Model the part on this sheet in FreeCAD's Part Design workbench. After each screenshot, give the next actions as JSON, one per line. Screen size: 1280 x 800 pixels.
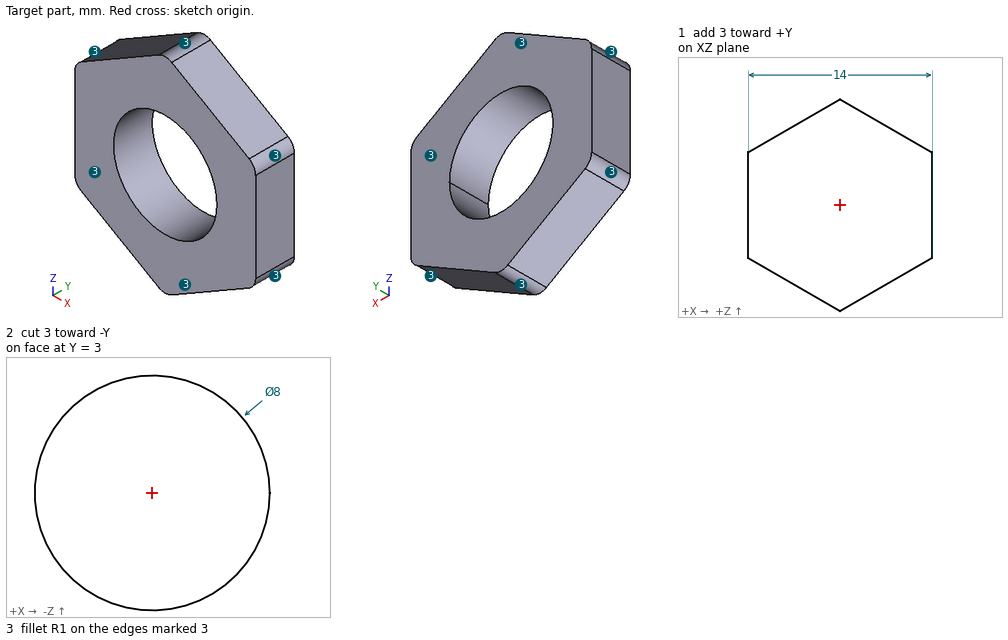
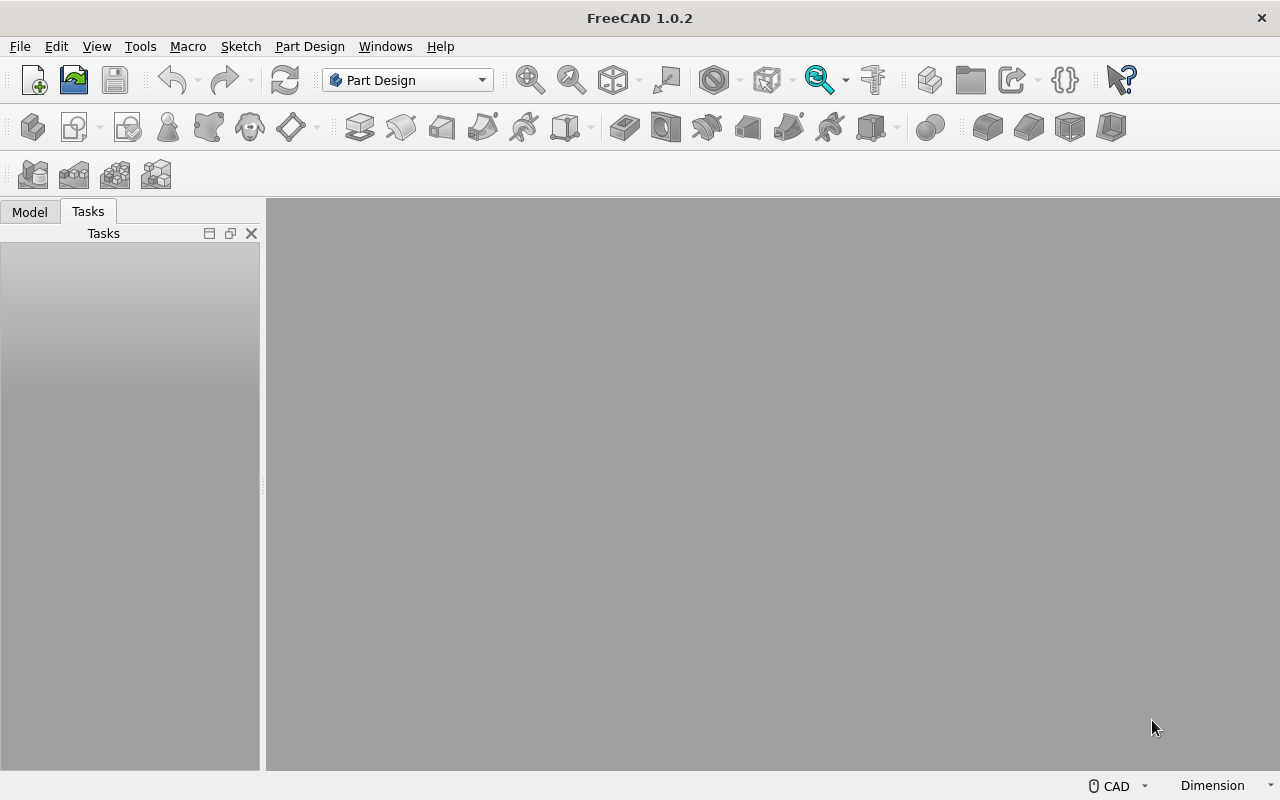
{"action": "key", "text": "ctrl+n"}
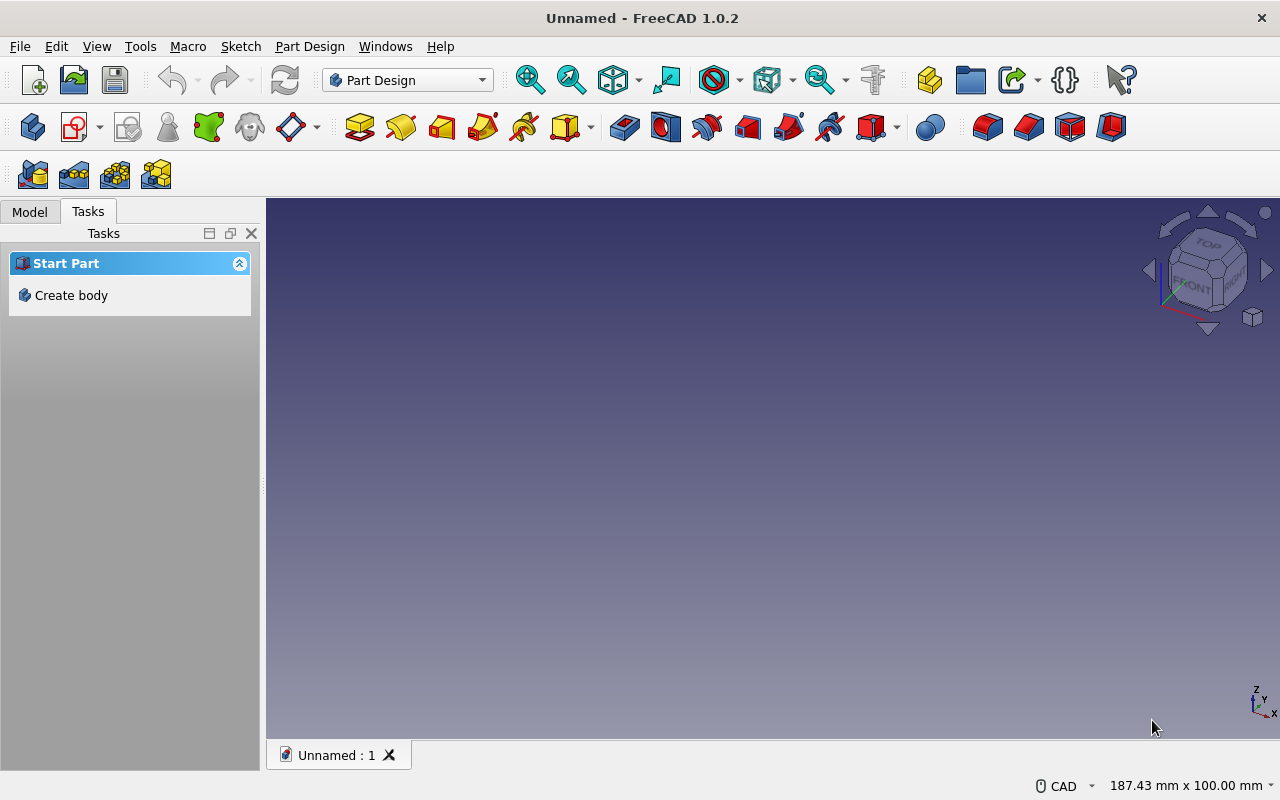
{"action": "left_click", "coordinate": [74, 128]}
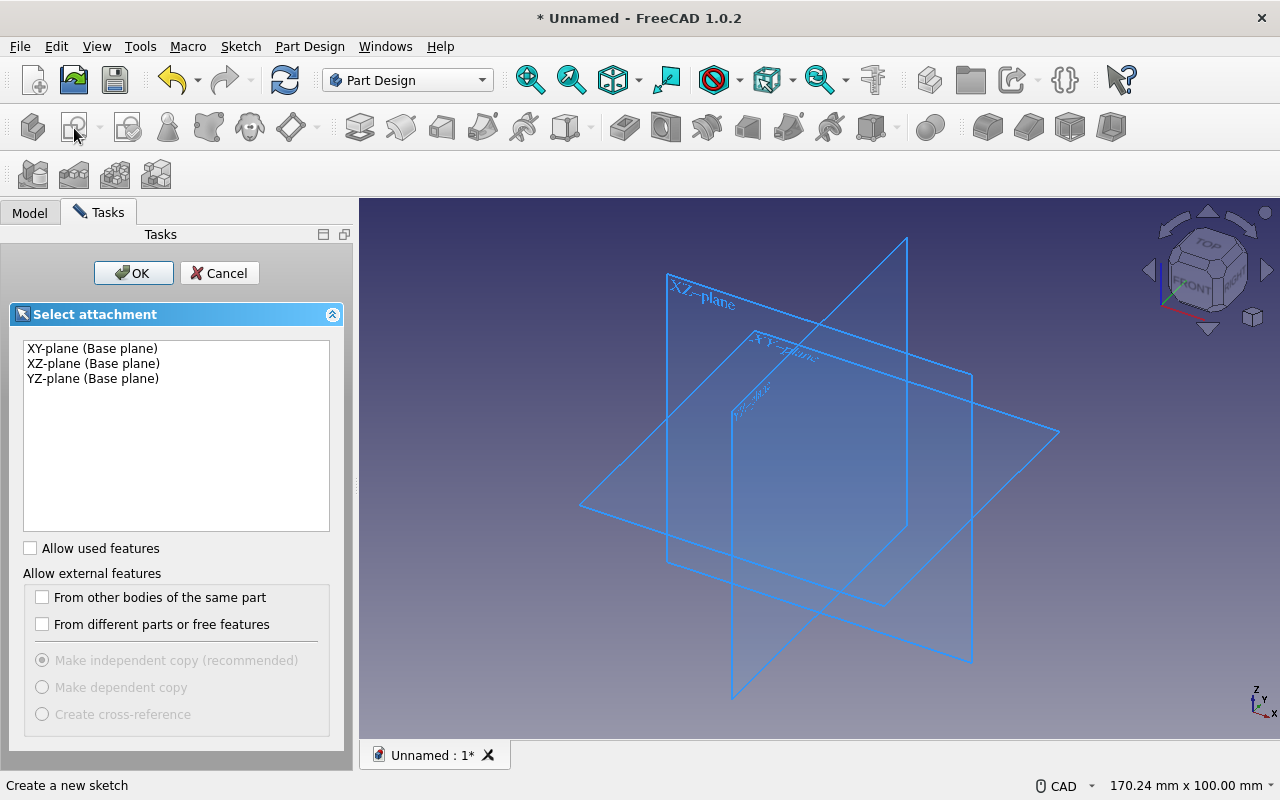
{"action": "left_click", "coordinate": [84, 364]}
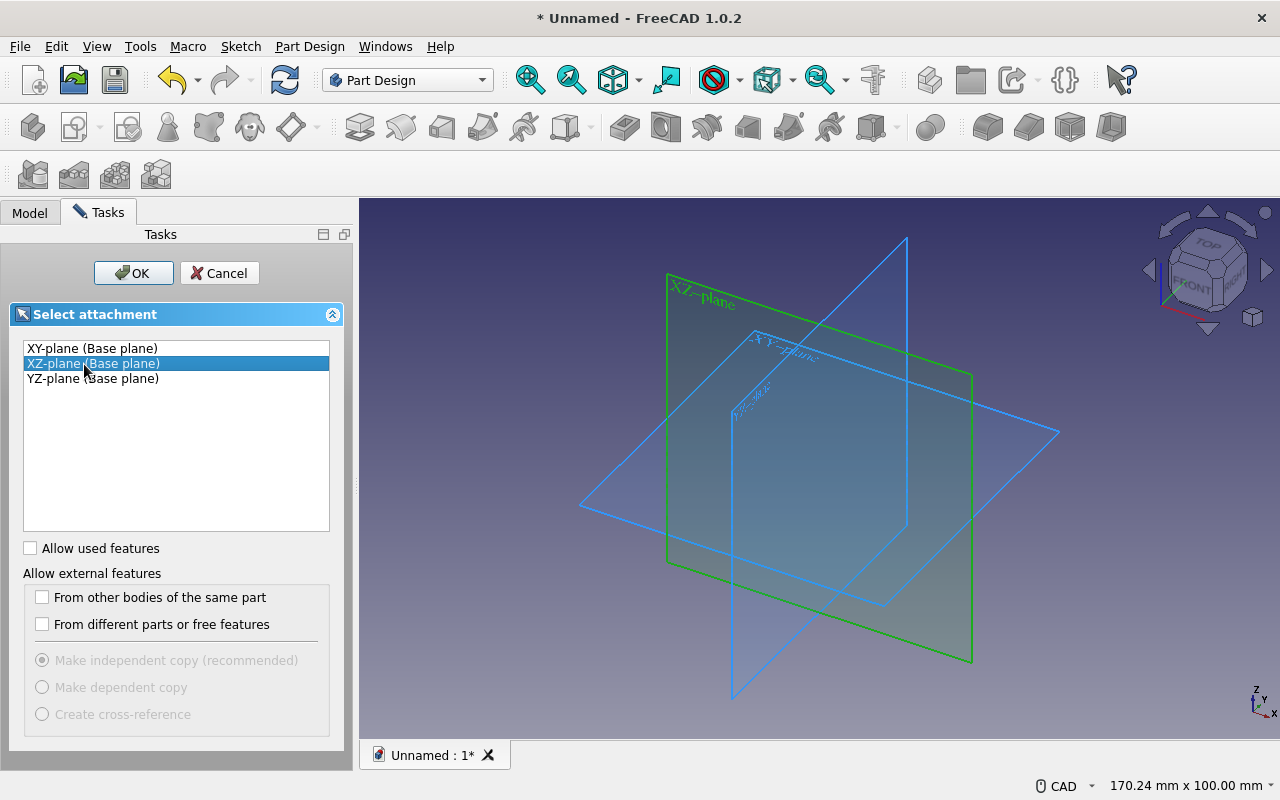
{"action": "left_click", "coordinate": [134, 273]}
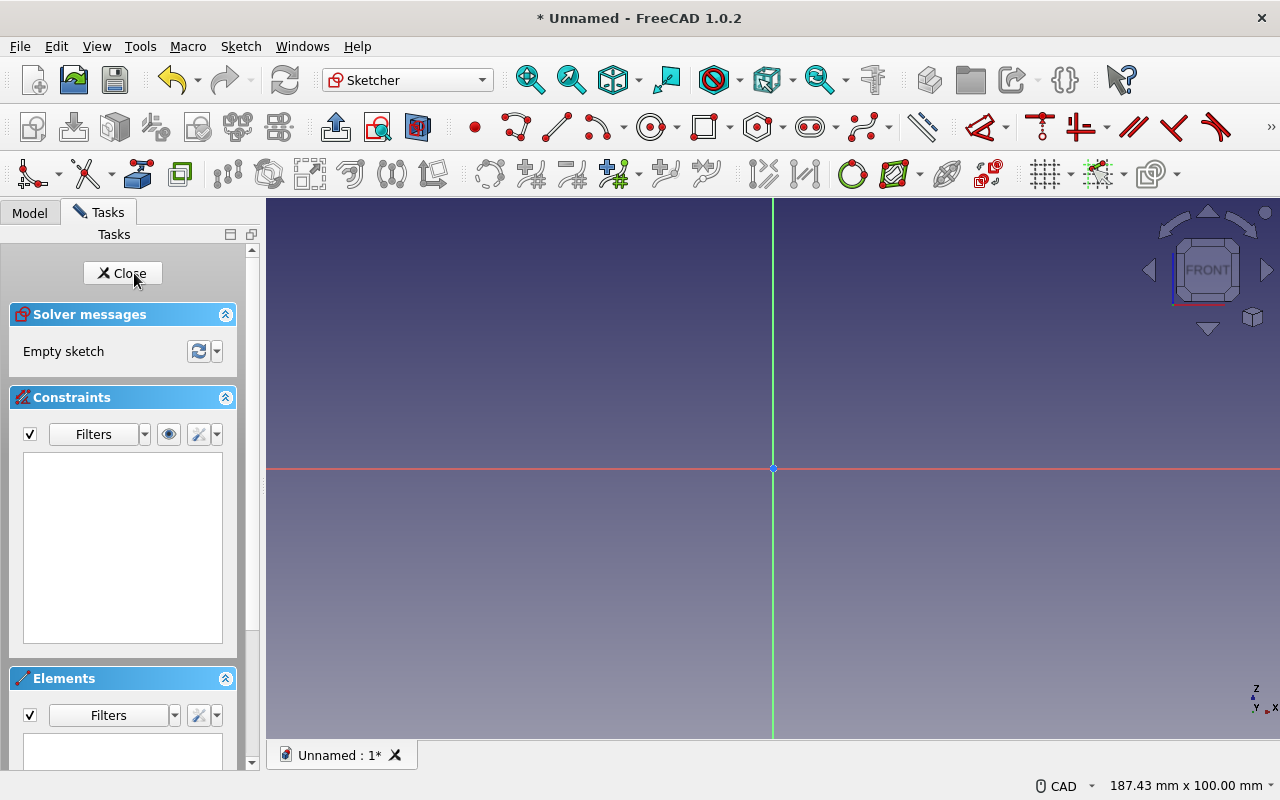
{"action": "scroll", "coordinate": [795, 468], "scroll_direction": "up", "scroll_amount": 7}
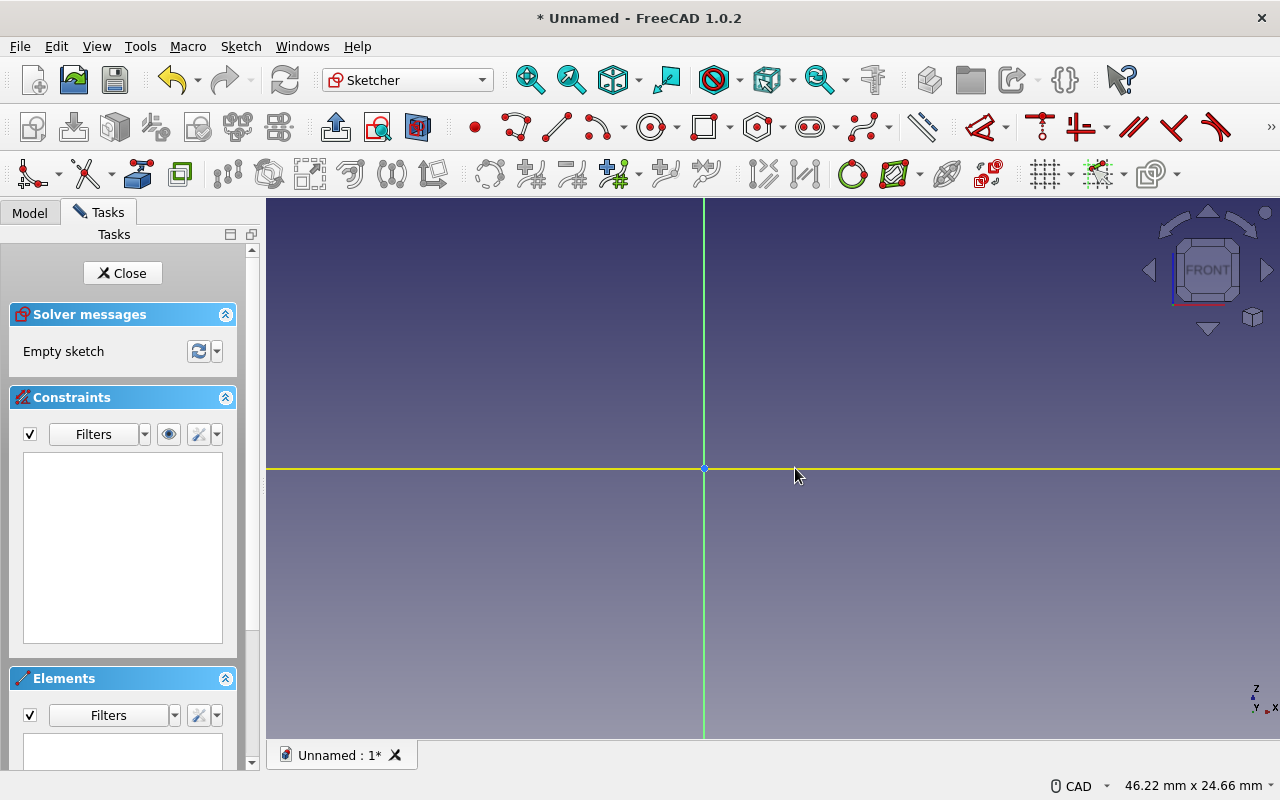
{"action": "key", "text": "g p 6"}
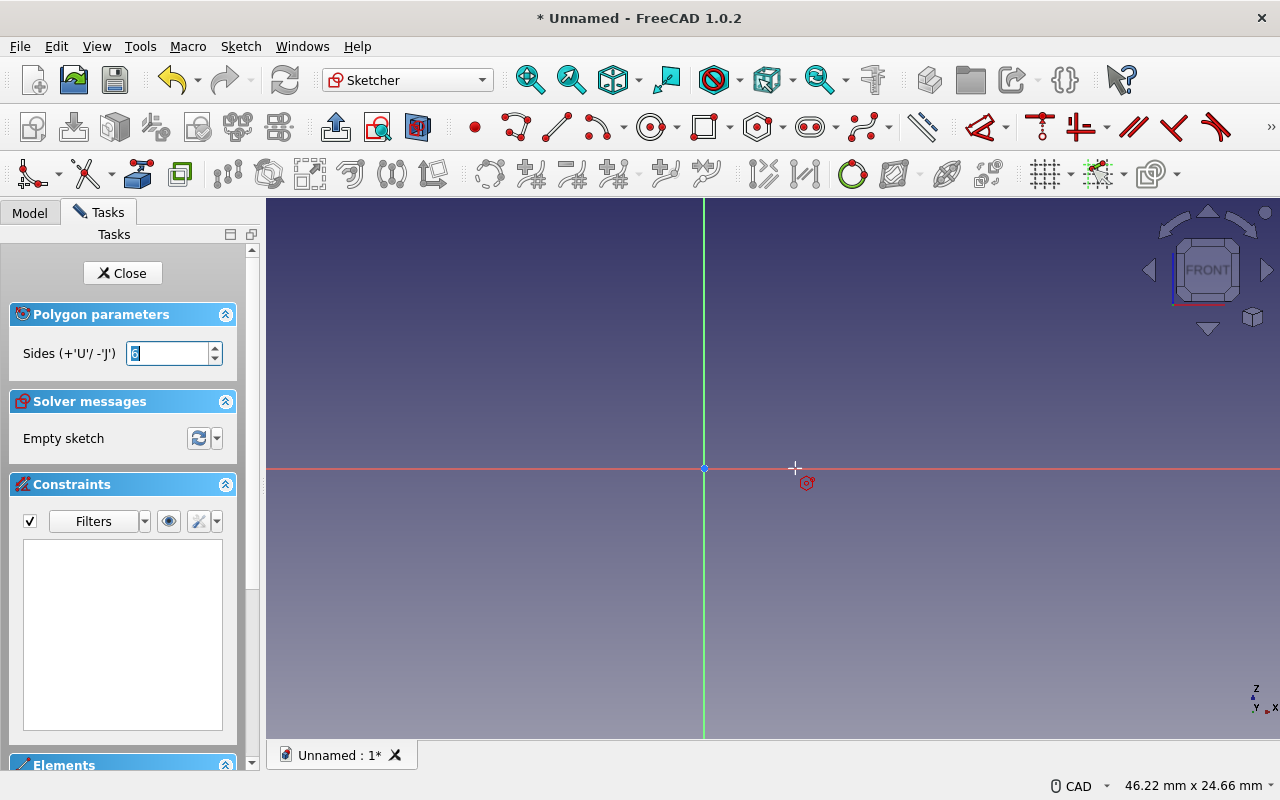
{"action": "left_click", "coordinate": [704, 468]}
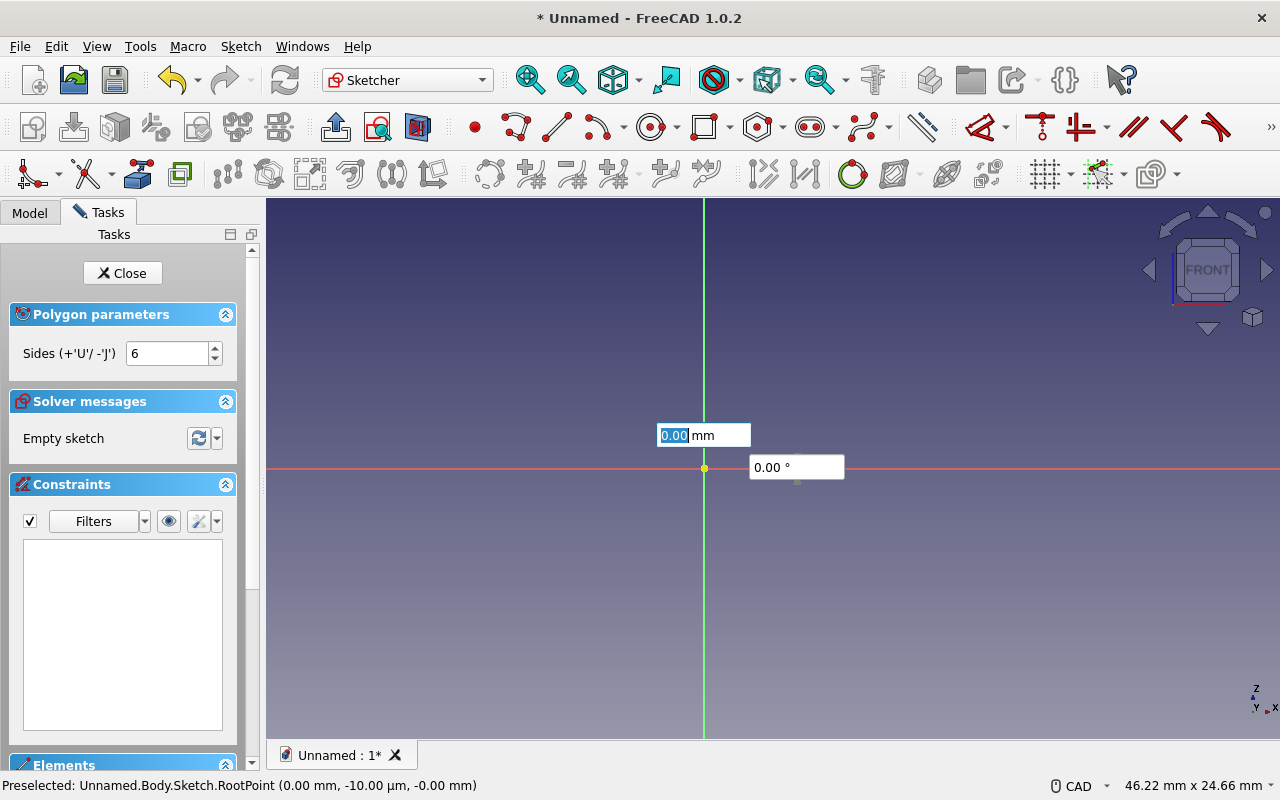
{"action": "left_click", "coordinate": [704, 646]}
{"action": "right_click", "coordinate": [704, 646]}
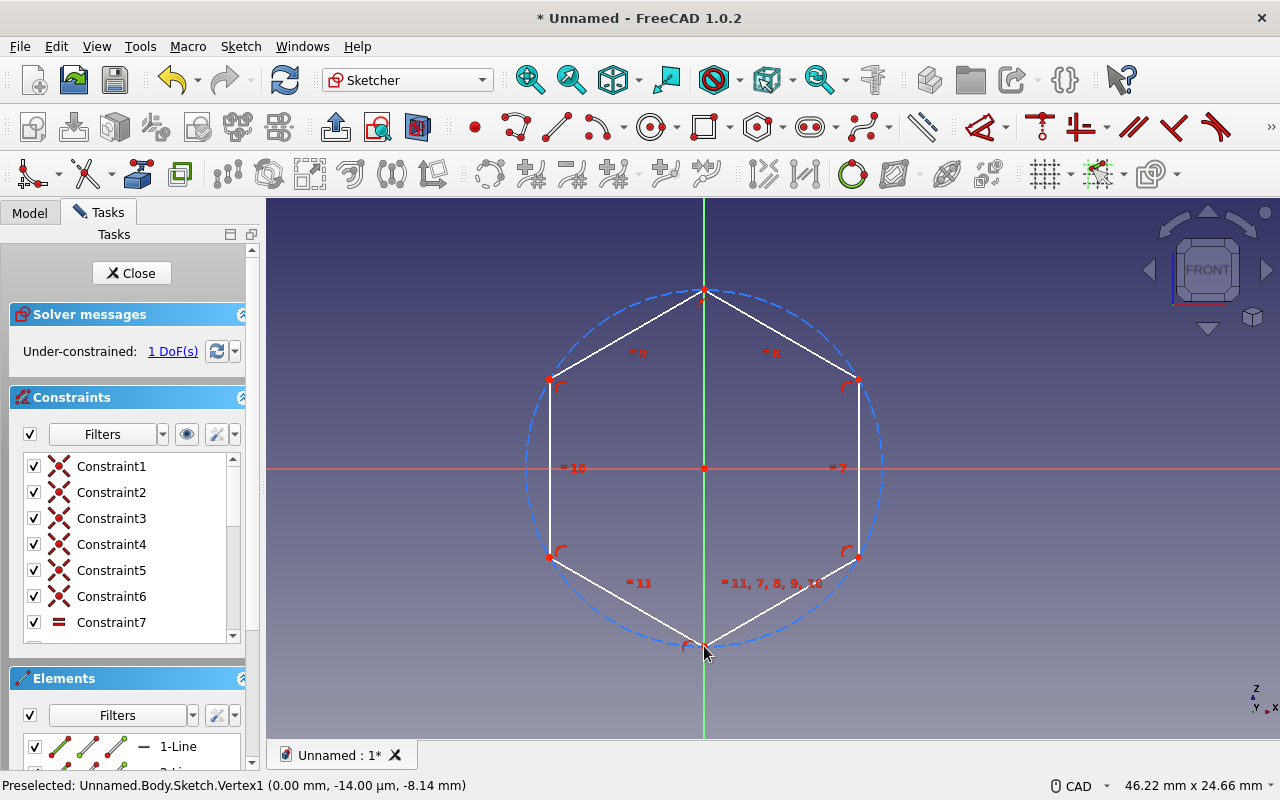
{"action": "left_click", "coordinate": [980, 128]}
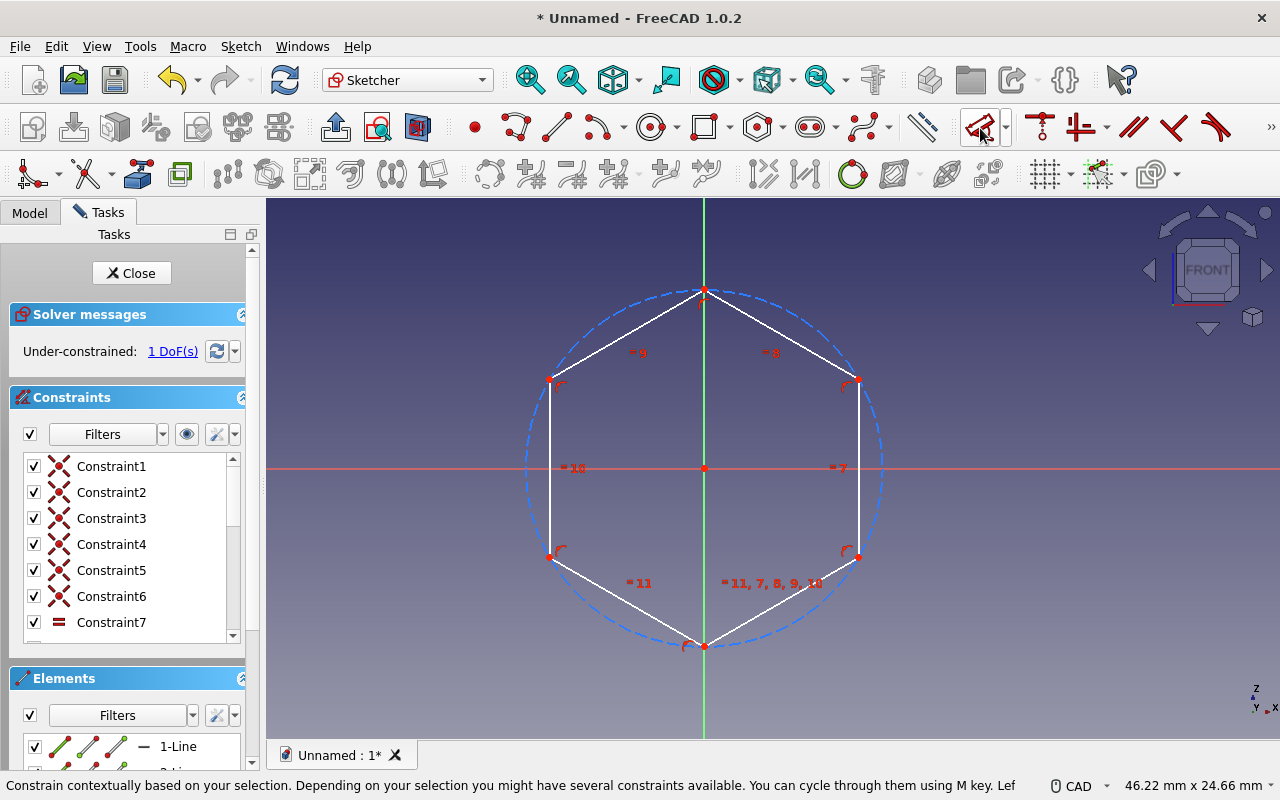
{"action": "left_click", "coordinate": [550, 379]}